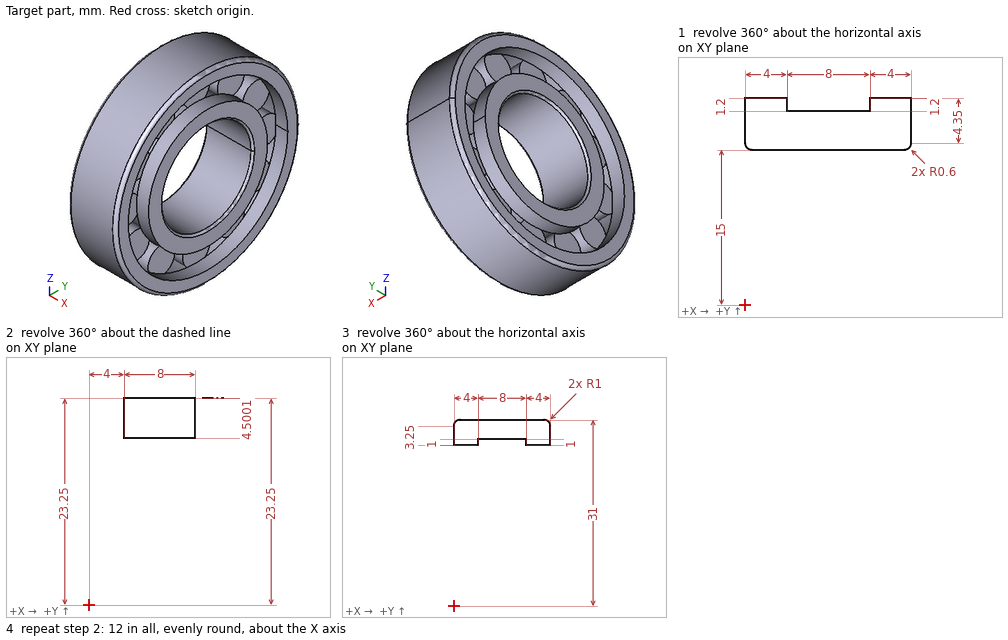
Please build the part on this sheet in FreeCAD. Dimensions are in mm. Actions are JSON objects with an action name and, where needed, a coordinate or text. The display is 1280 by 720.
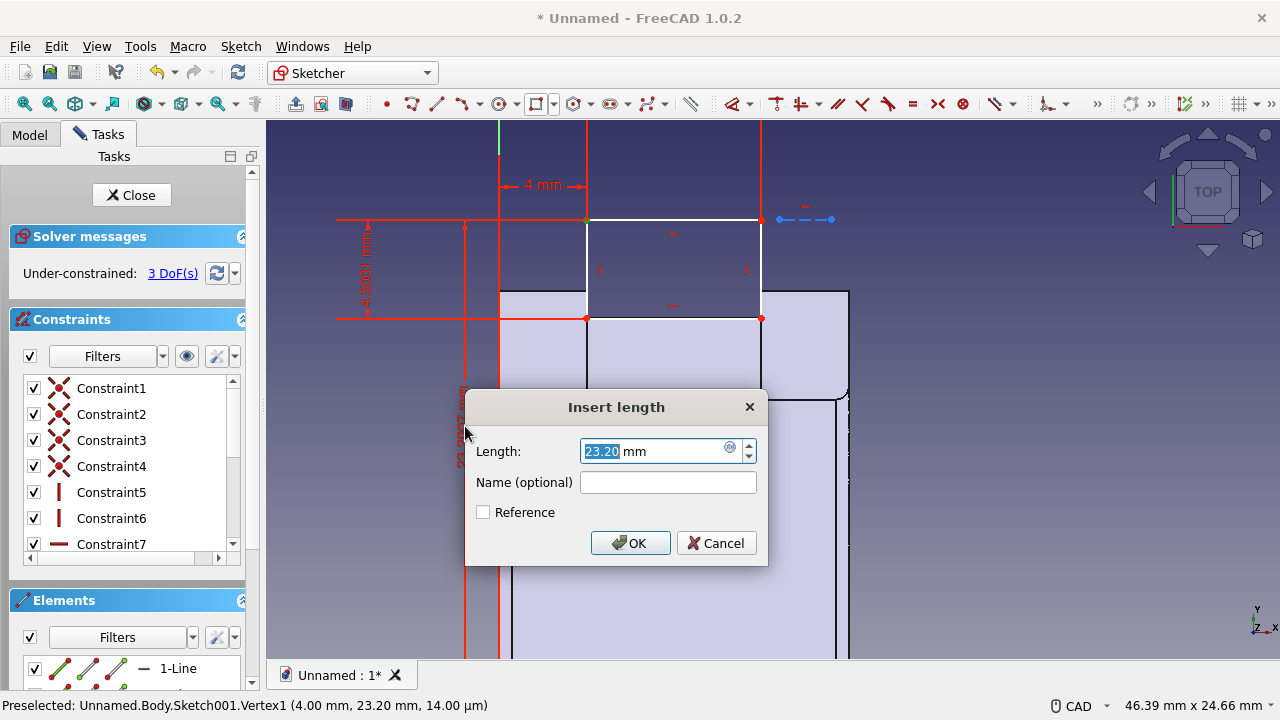
{"action": "type", "text": "23.25"}
{"action": "key", "text": "Return"}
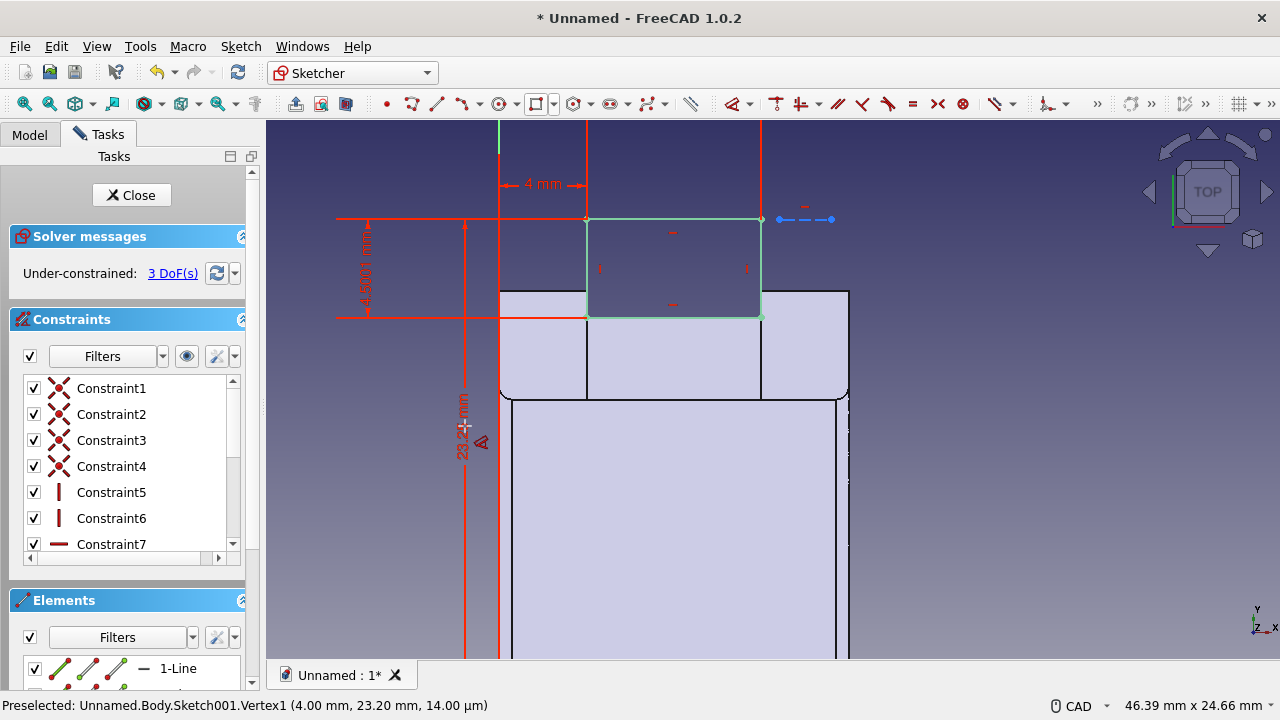
{"action": "left_click", "coordinate": [779, 220]}
{"action": "left_click", "coordinate": [465, 331]}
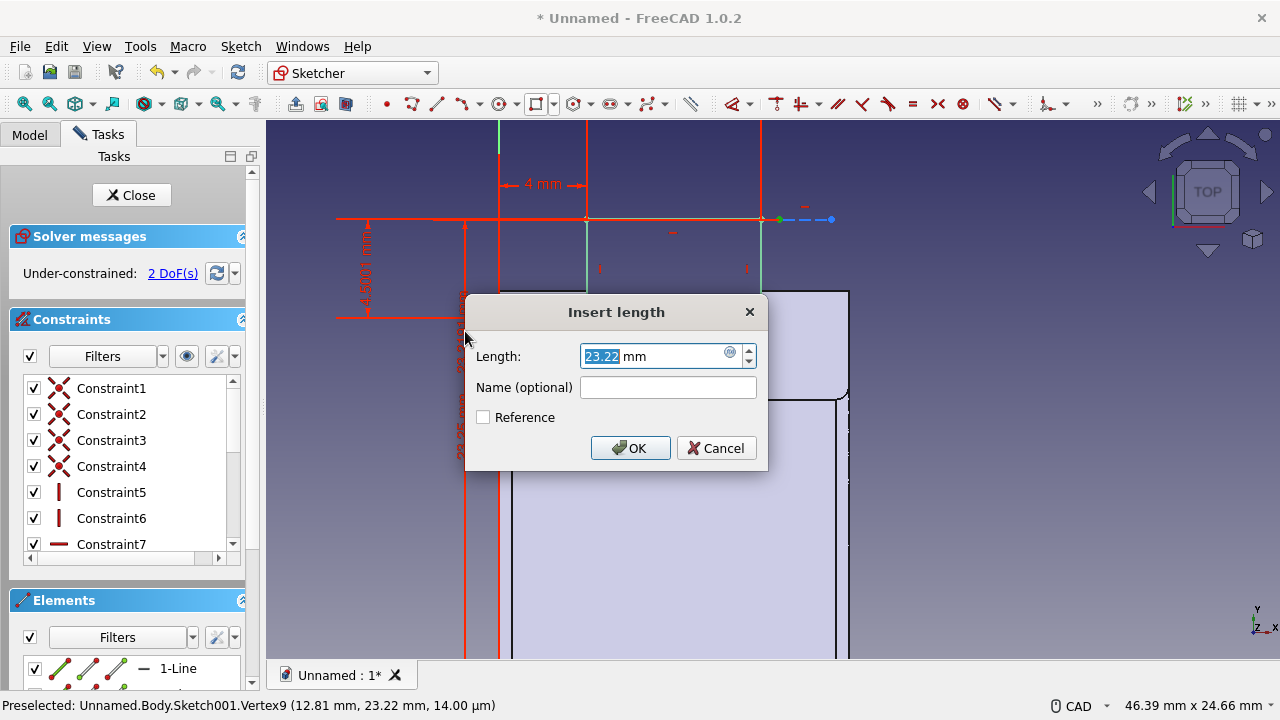
{"action": "type", "text": "23.25"}
{"action": "key", "text": "Return"}
{"action": "key", "text": "Escape"}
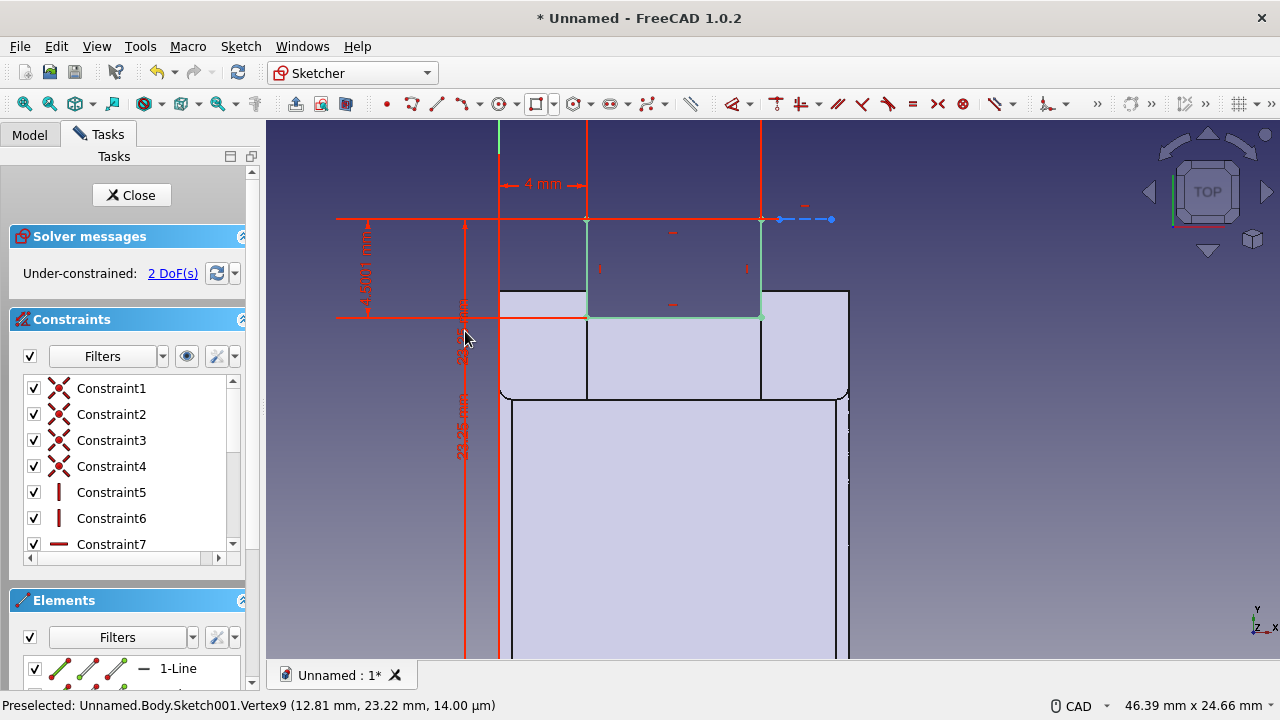
{"action": "left_click", "coordinate": [132, 195]}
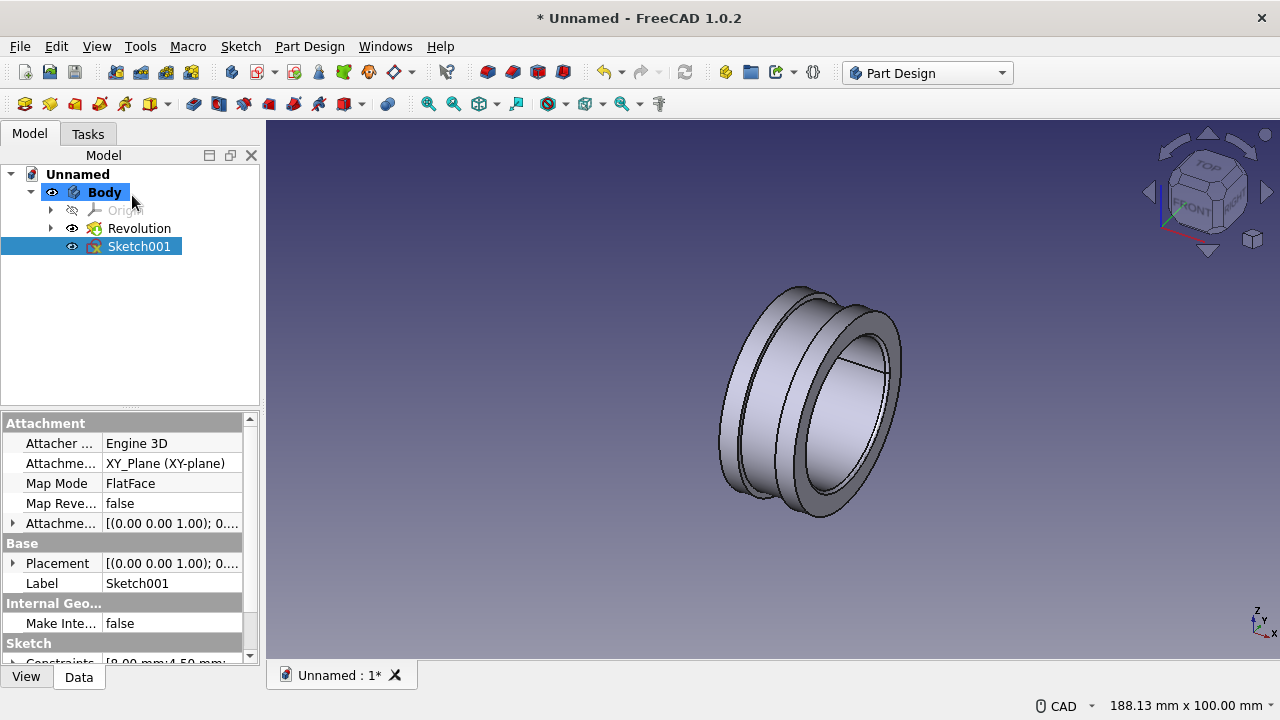
{"action": "left_click", "coordinate": [50, 104]}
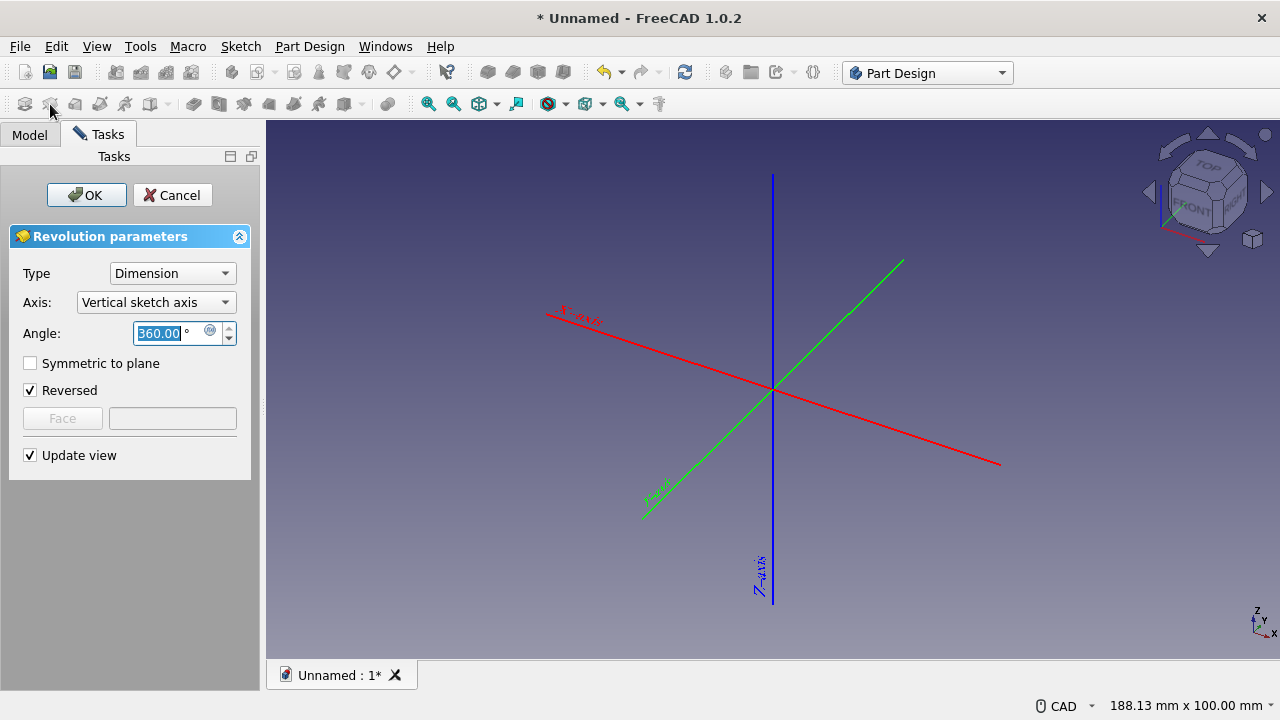
{"action": "left_click", "coordinate": [157, 302]}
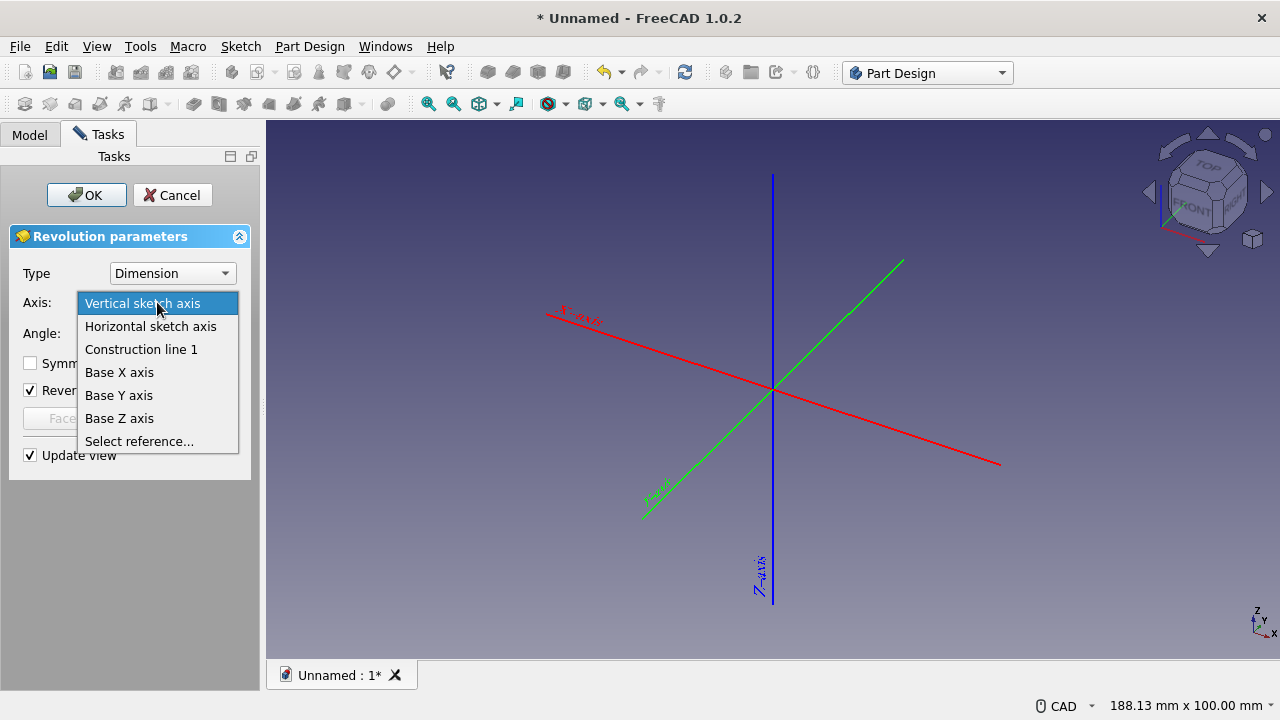
{"action": "left_click", "coordinate": [156, 350]}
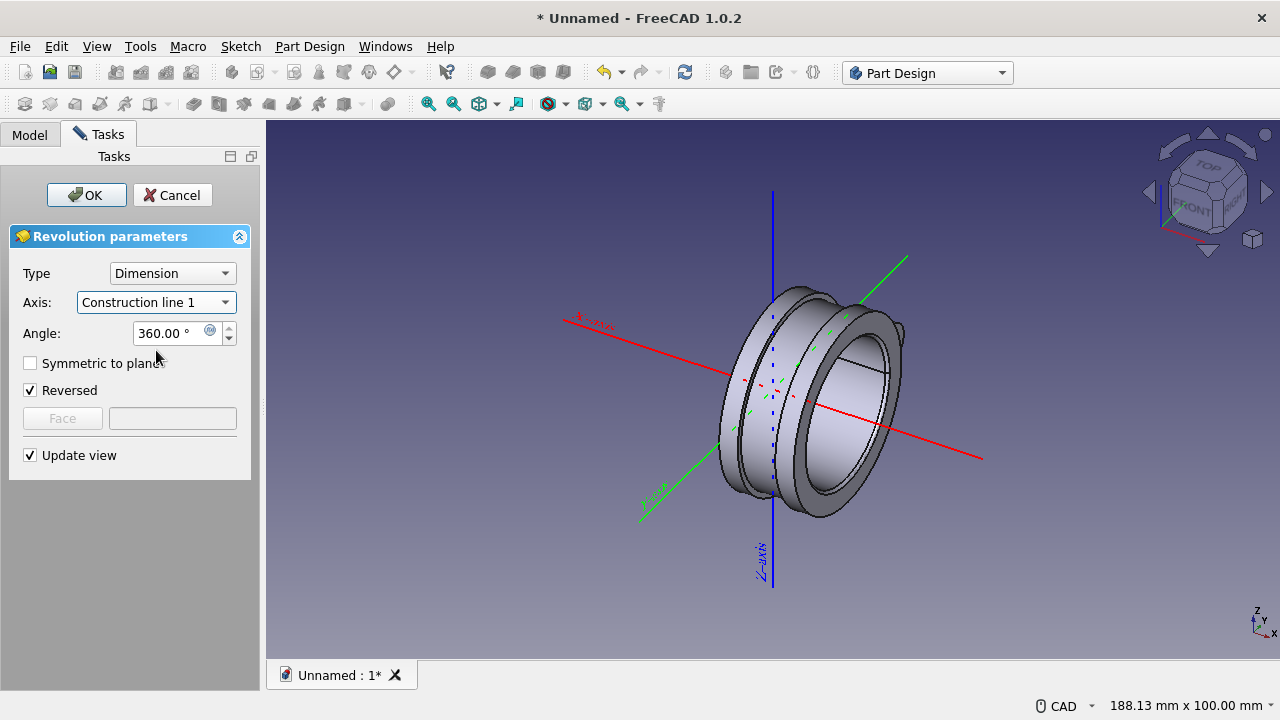
{"action": "left_click", "coordinate": [87, 195]}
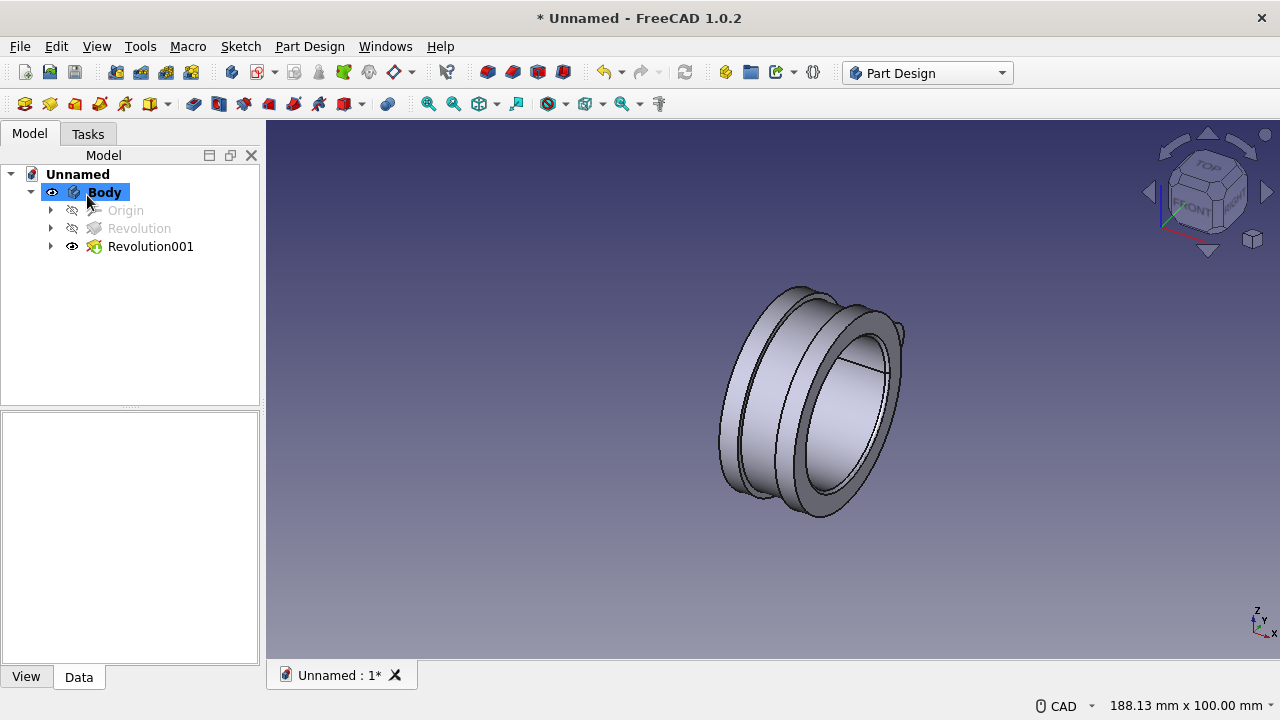
{"action": "left_click", "coordinate": [256, 72]}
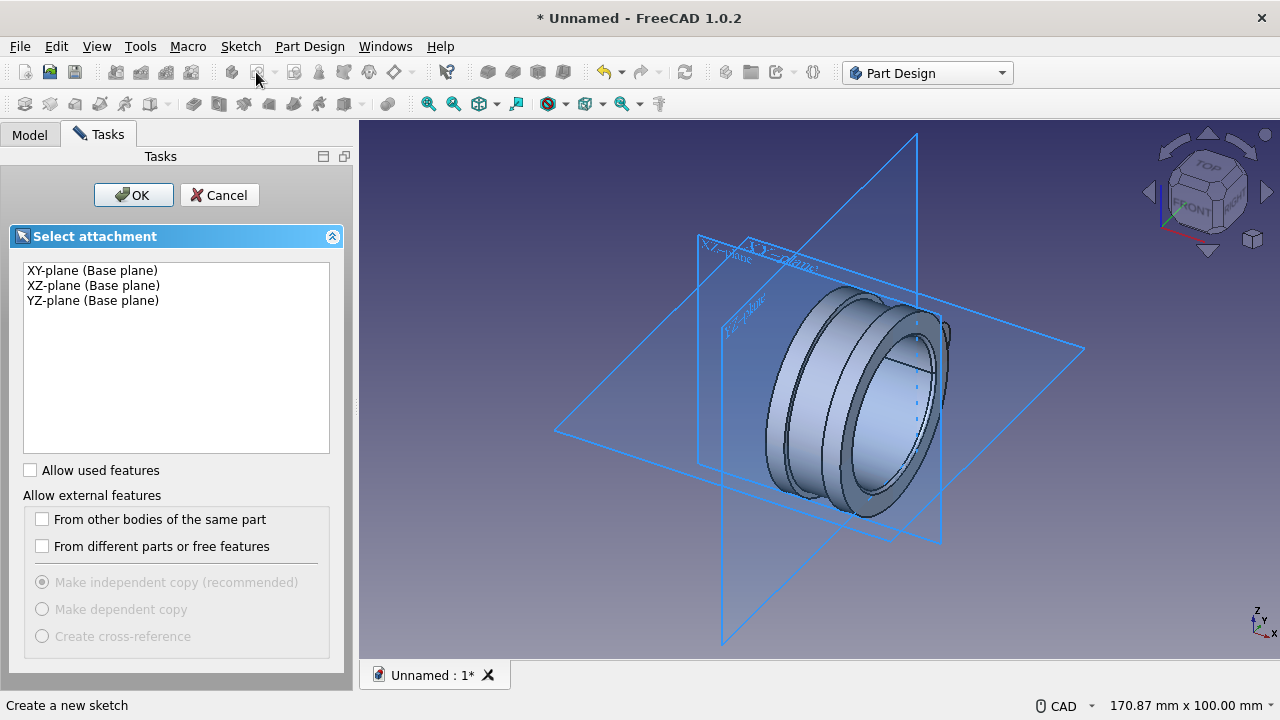
{"action": "left_click", "coordinate": [84, 270]}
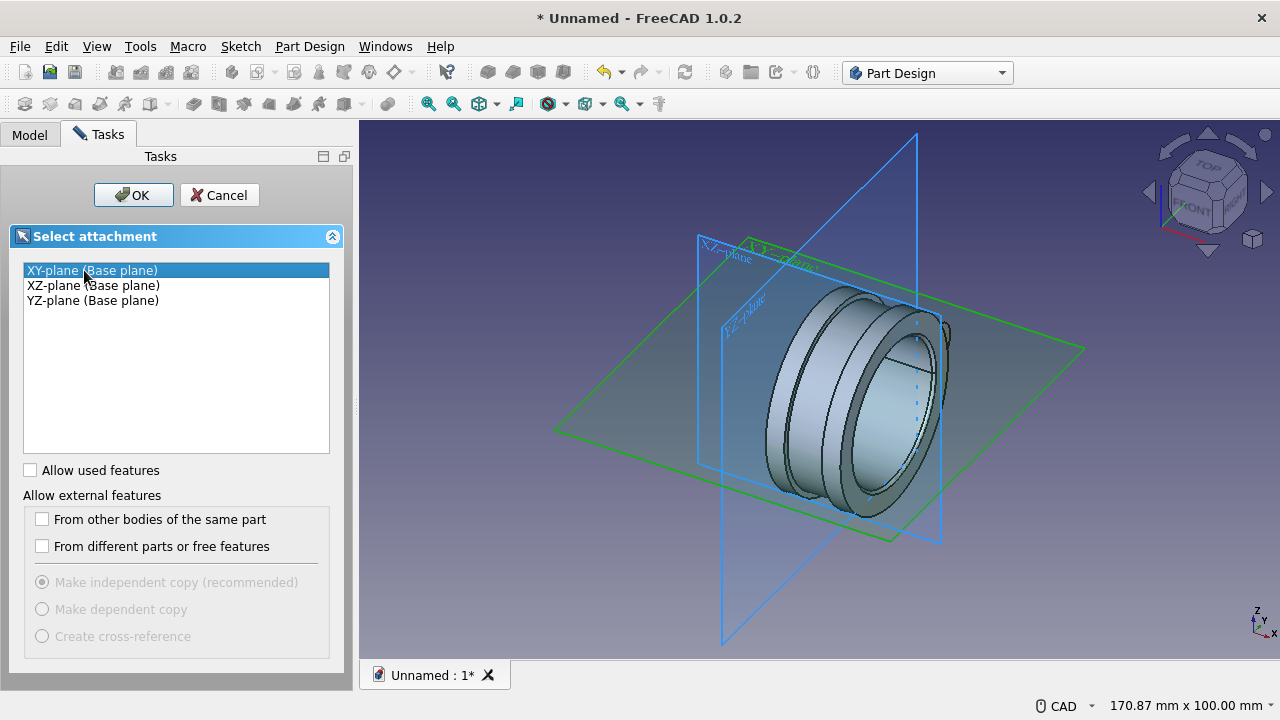
{"action": "left_click", "coordinate": [134, 195]}